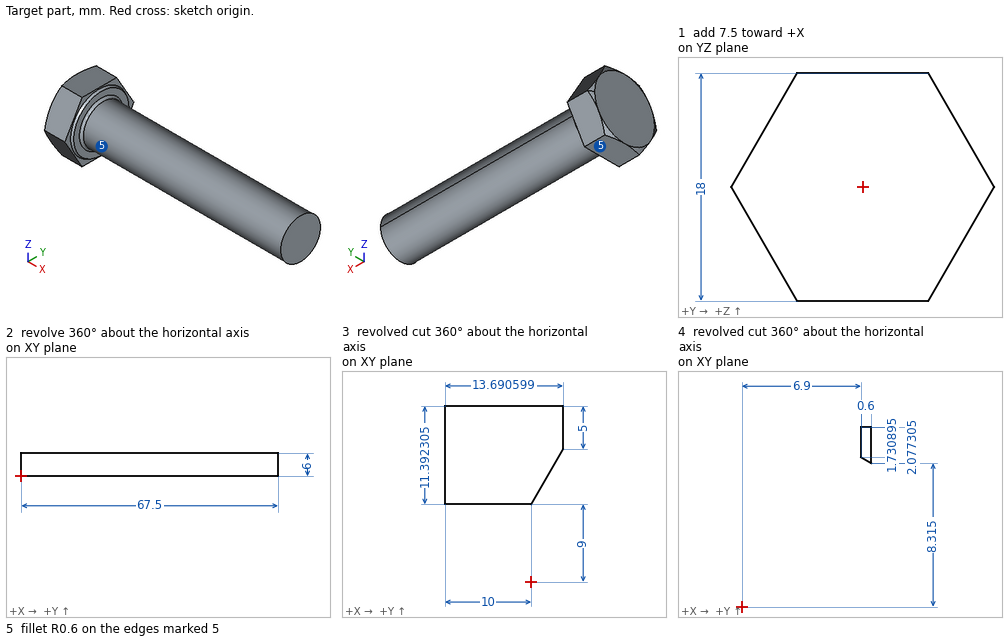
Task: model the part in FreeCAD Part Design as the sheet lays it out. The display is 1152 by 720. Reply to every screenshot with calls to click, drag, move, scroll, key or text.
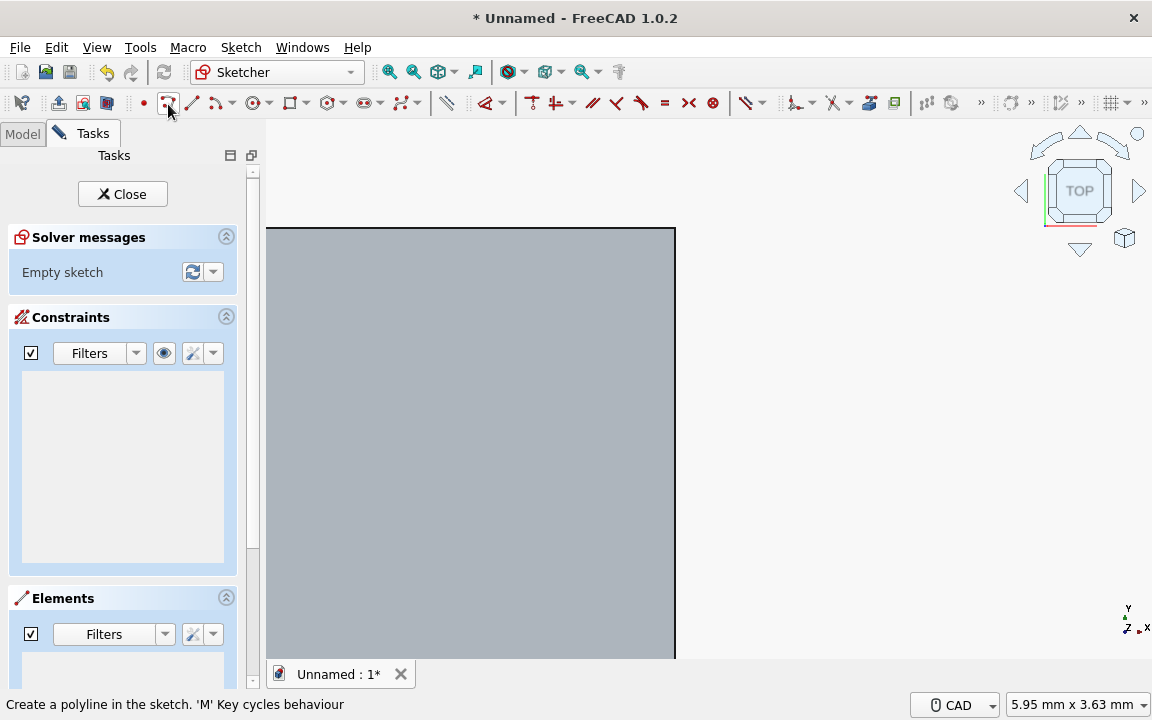
click(586, 486)
click(675, 537)
click(675, 228)
click(586, 228)
click(586, 487)
key(Escape)
key(Escape)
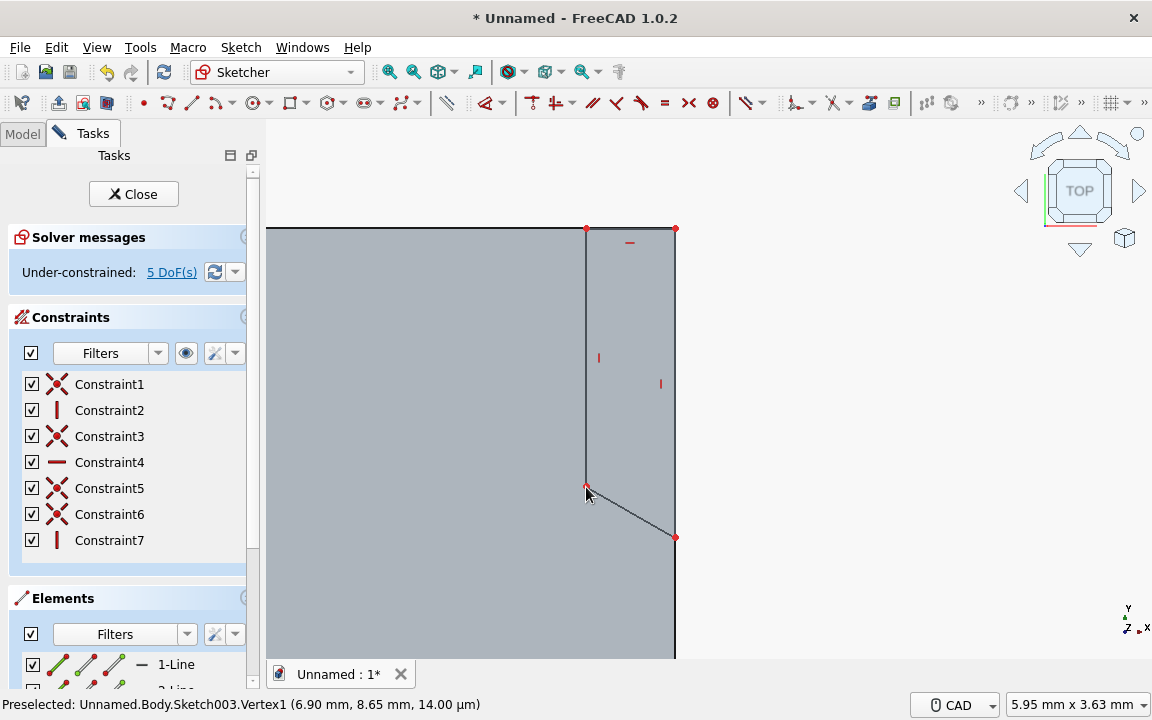
key(d)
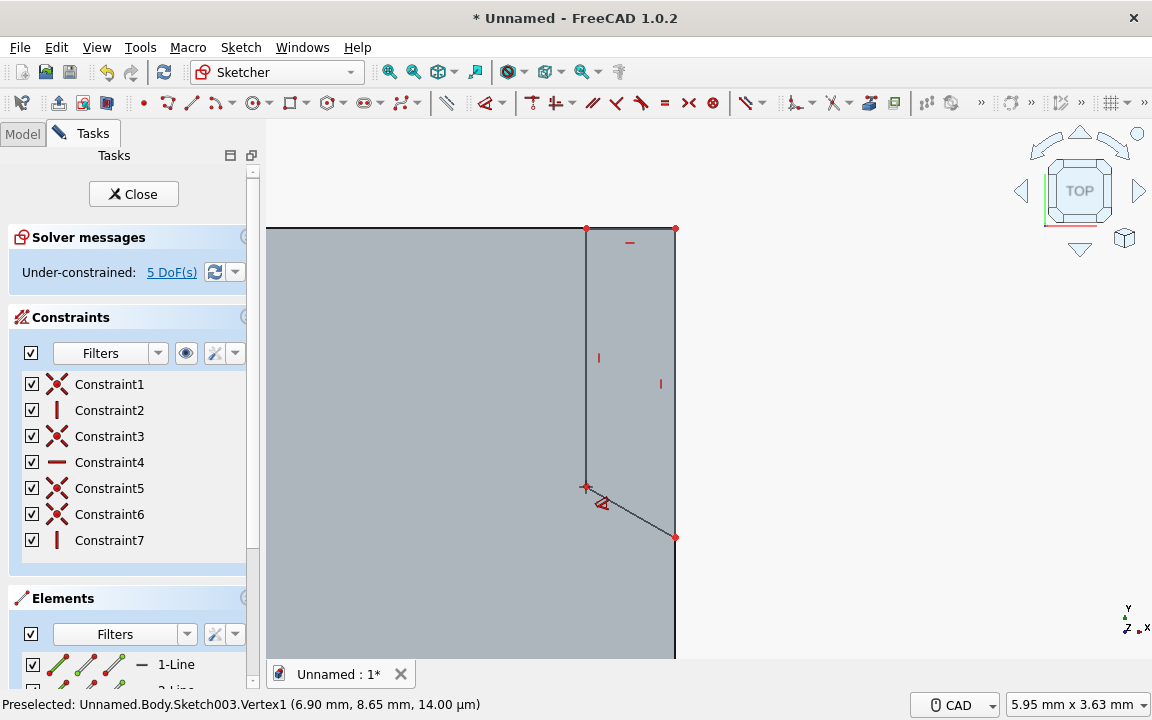
click(648, 229)
click(631, 195)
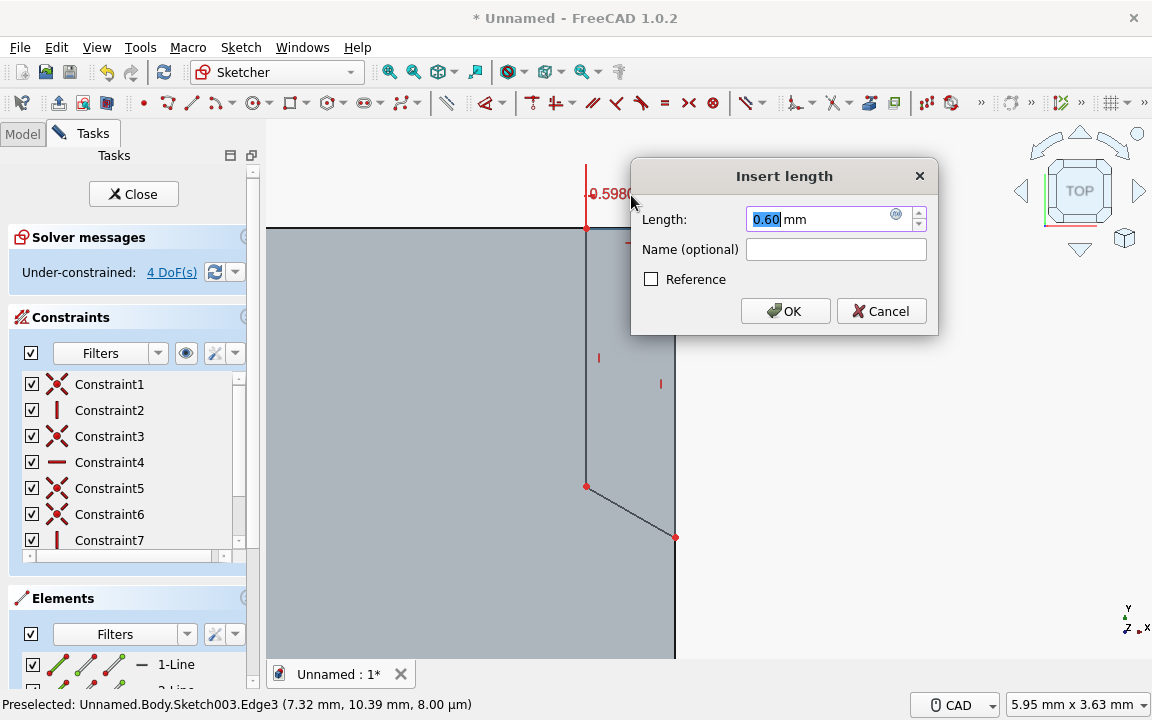
text(0.6)
key(Return)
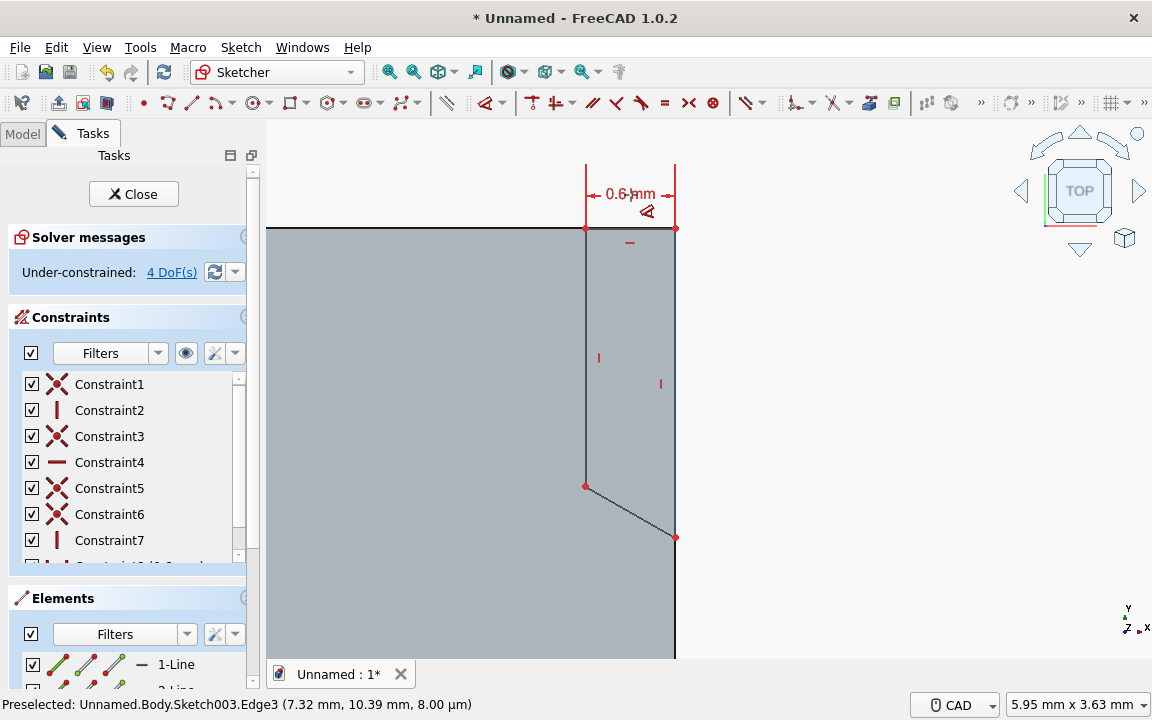
click(586, 487)
click(440, 453)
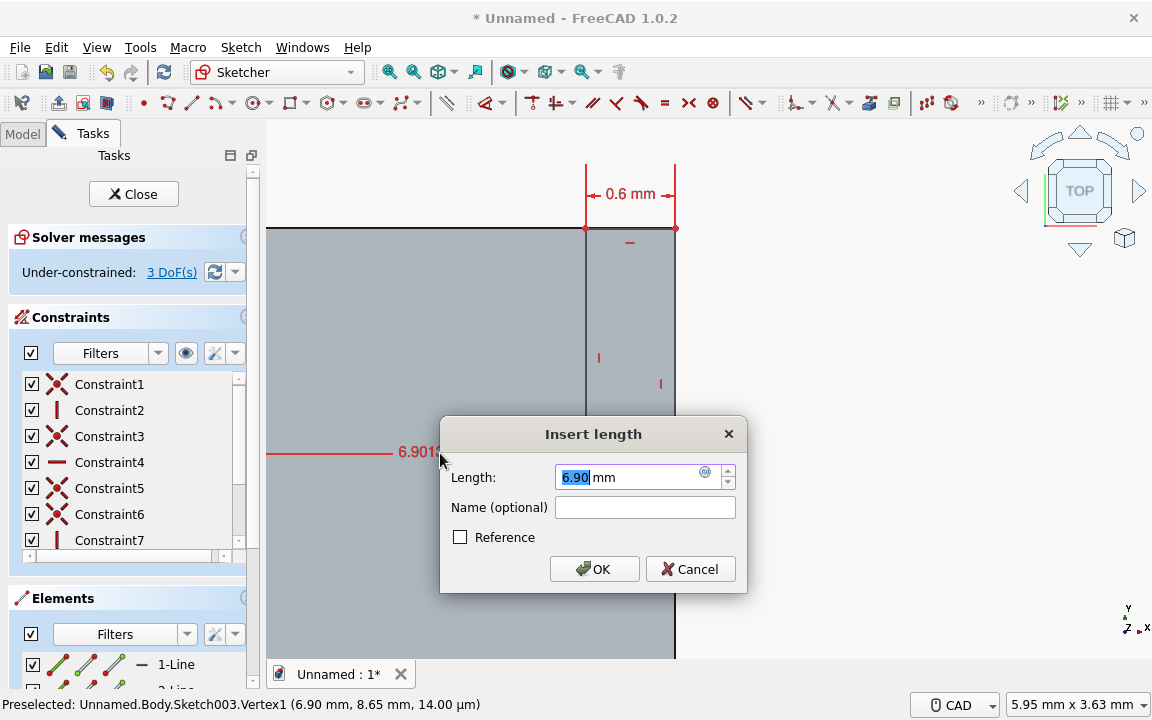
text(6.9)
key(Return)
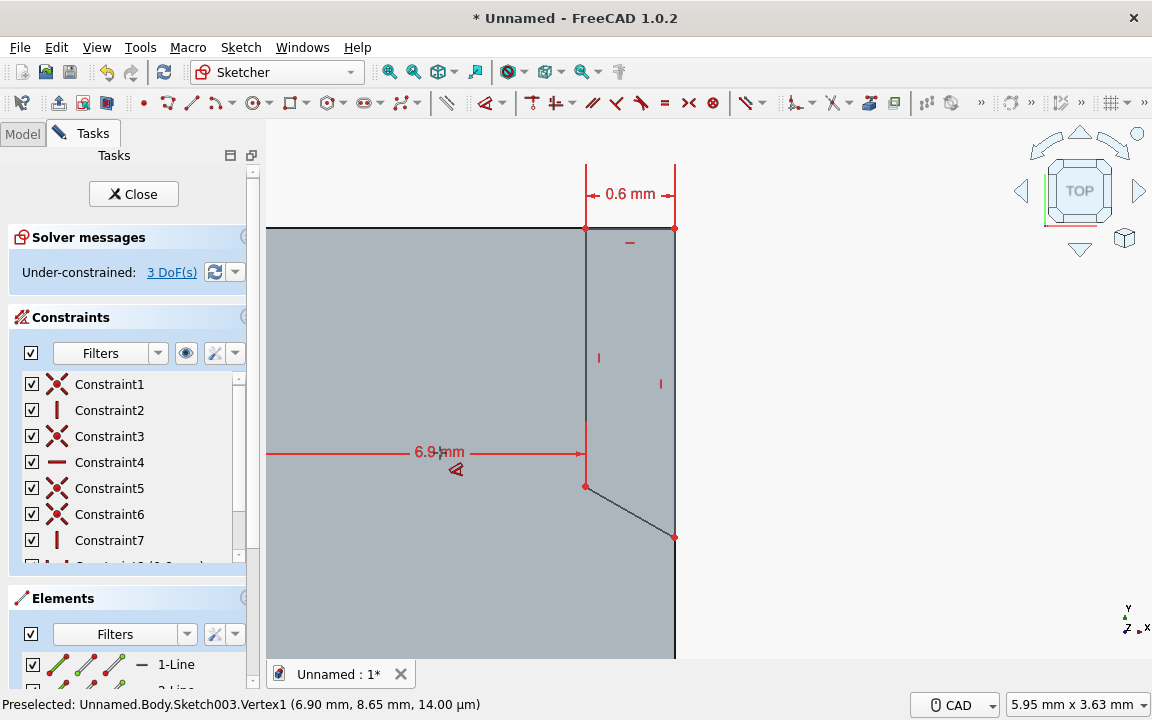
click(675, 538)
click(709, 585)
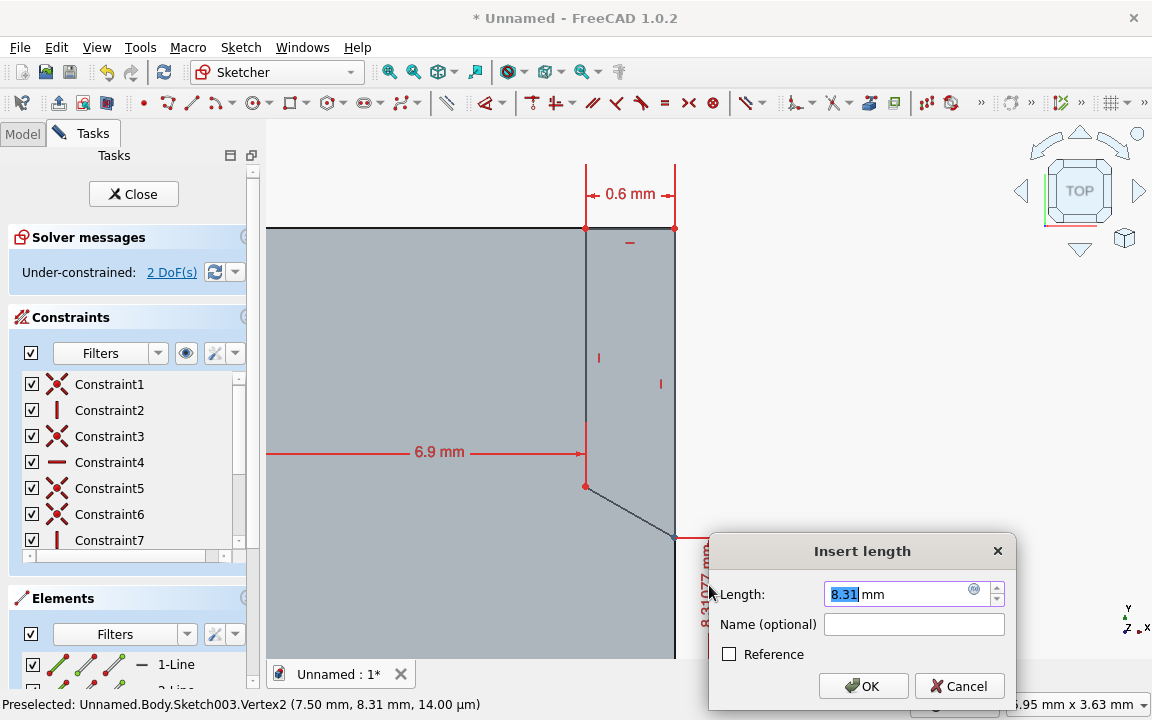
text(8.315)
key(Return)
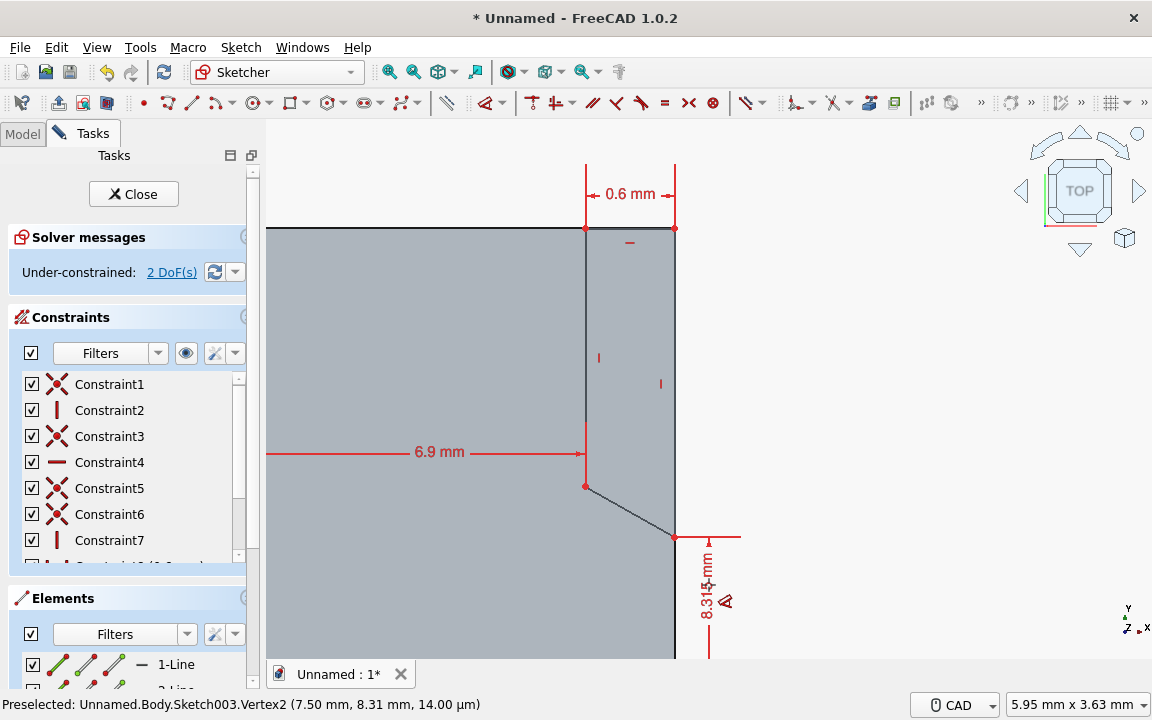
click(675, 445)
click(709, 383)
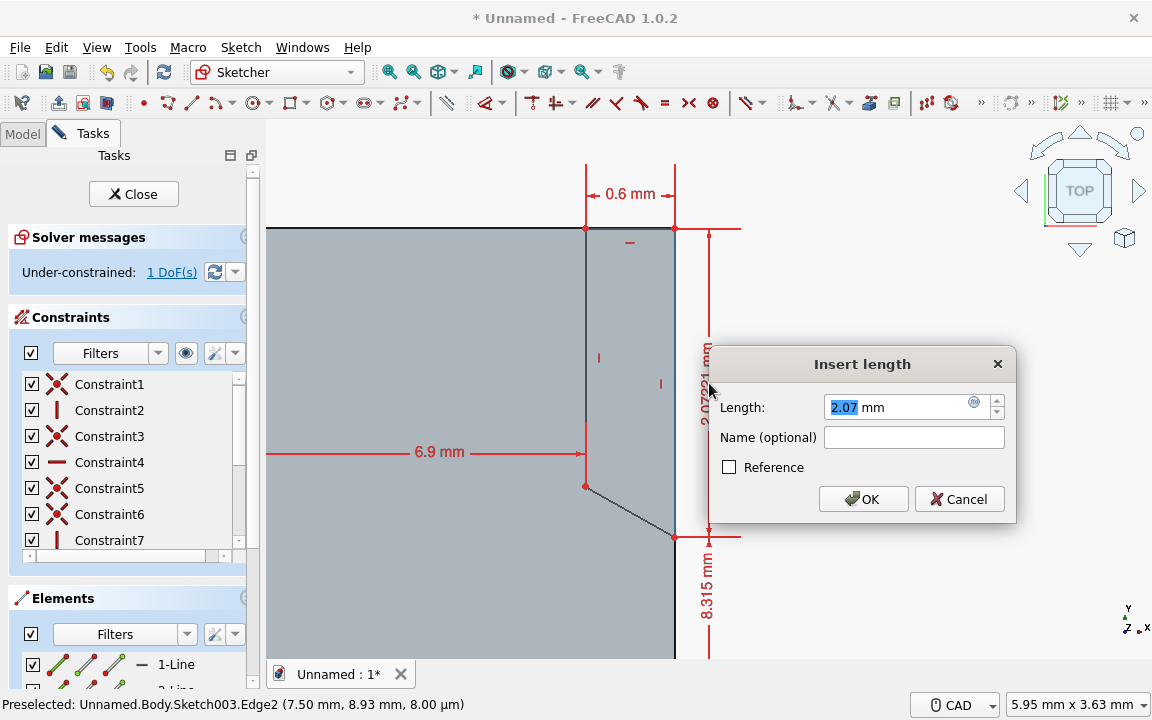
text(2.077305)
key(Return)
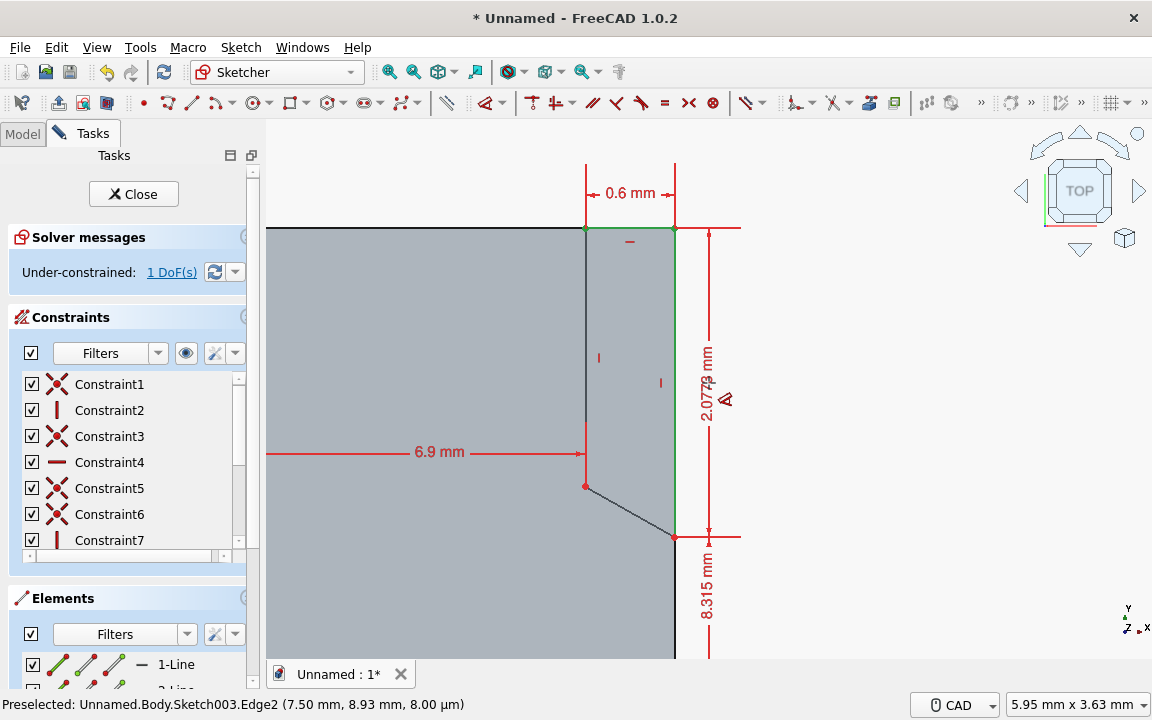
click(586, 306)
click(552, 358)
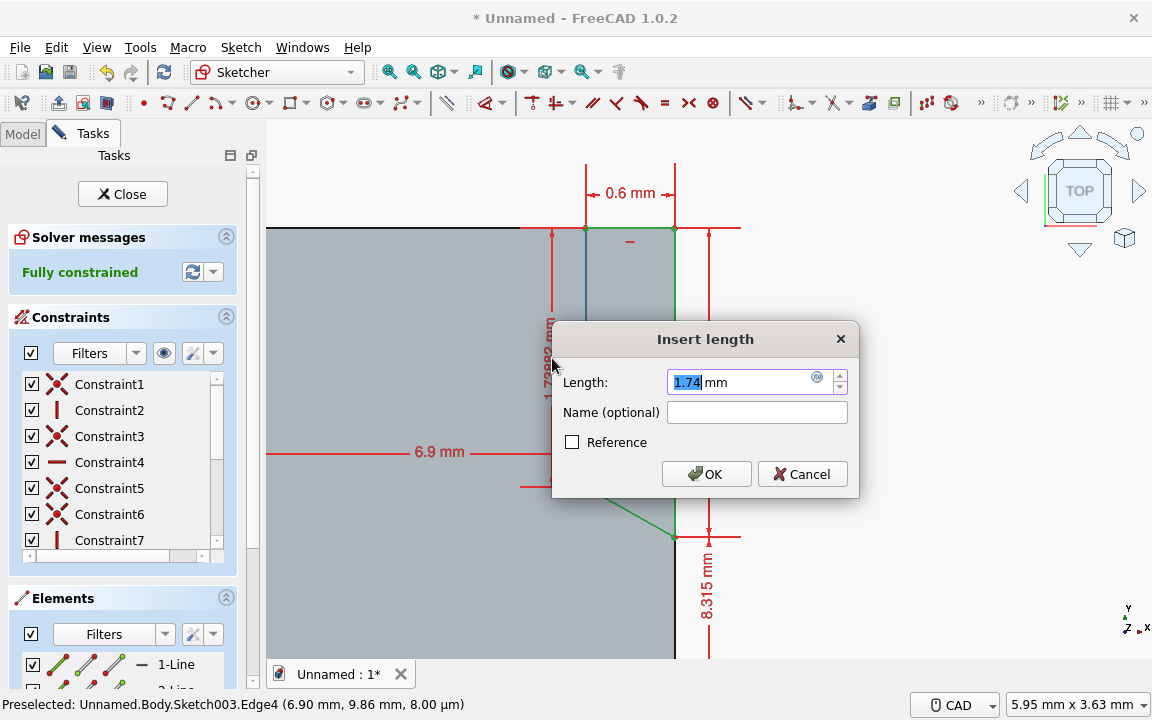
text(1.730895)
key(Return)
key(Escape)